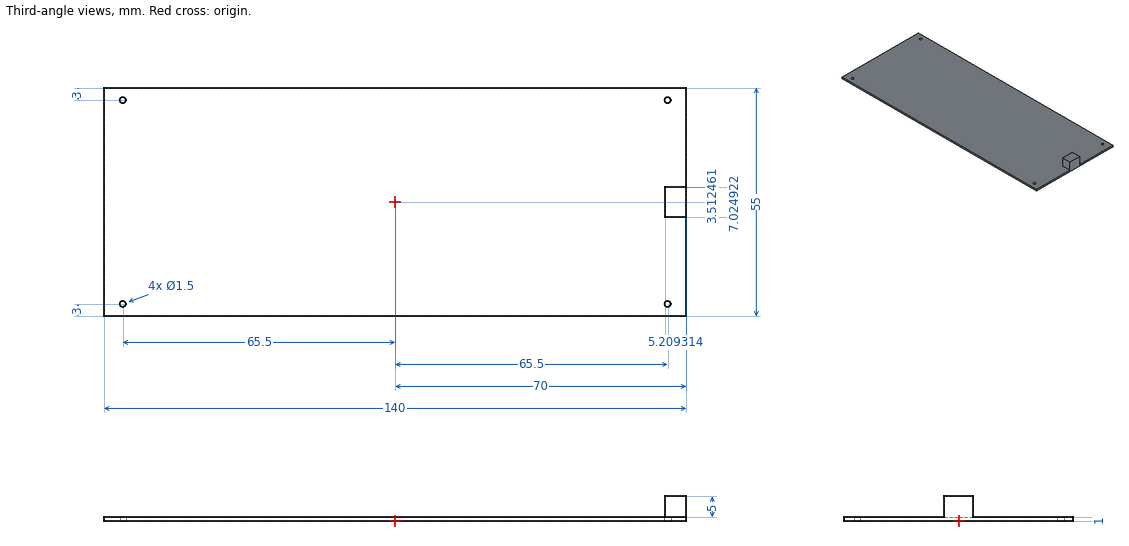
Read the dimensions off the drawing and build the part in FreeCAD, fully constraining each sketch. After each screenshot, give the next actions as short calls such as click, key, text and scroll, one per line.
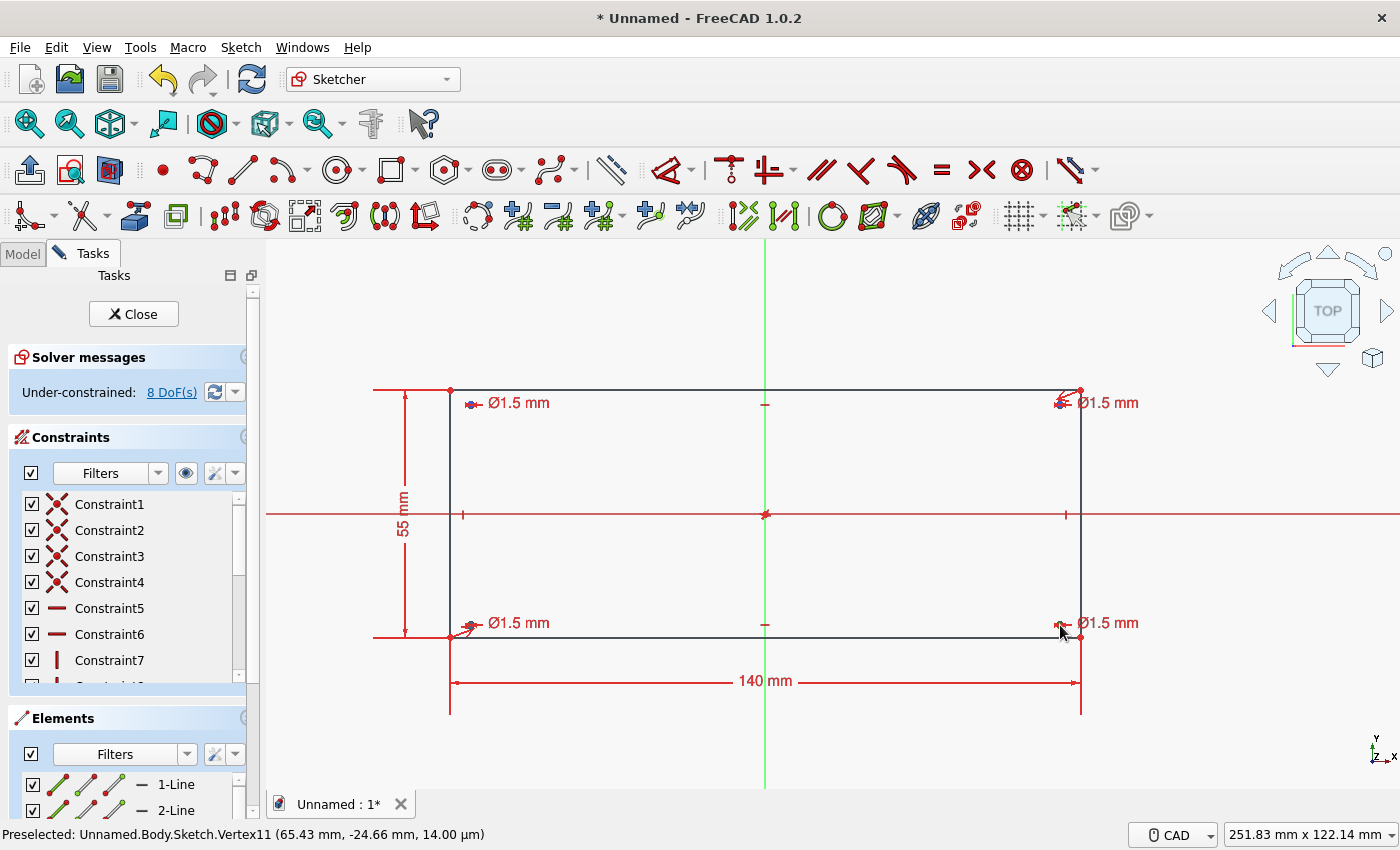
click(796, 170)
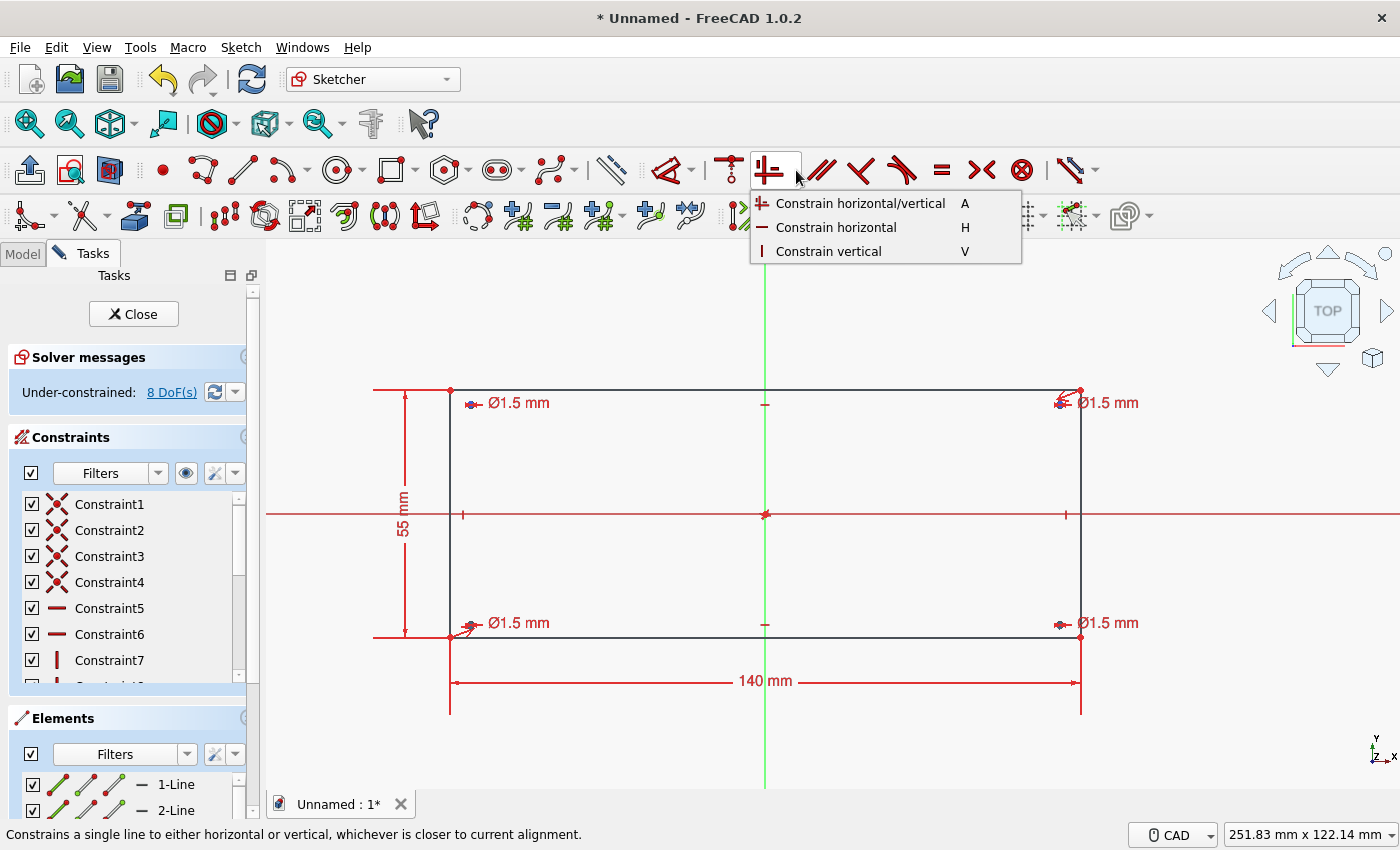
click(886, 227)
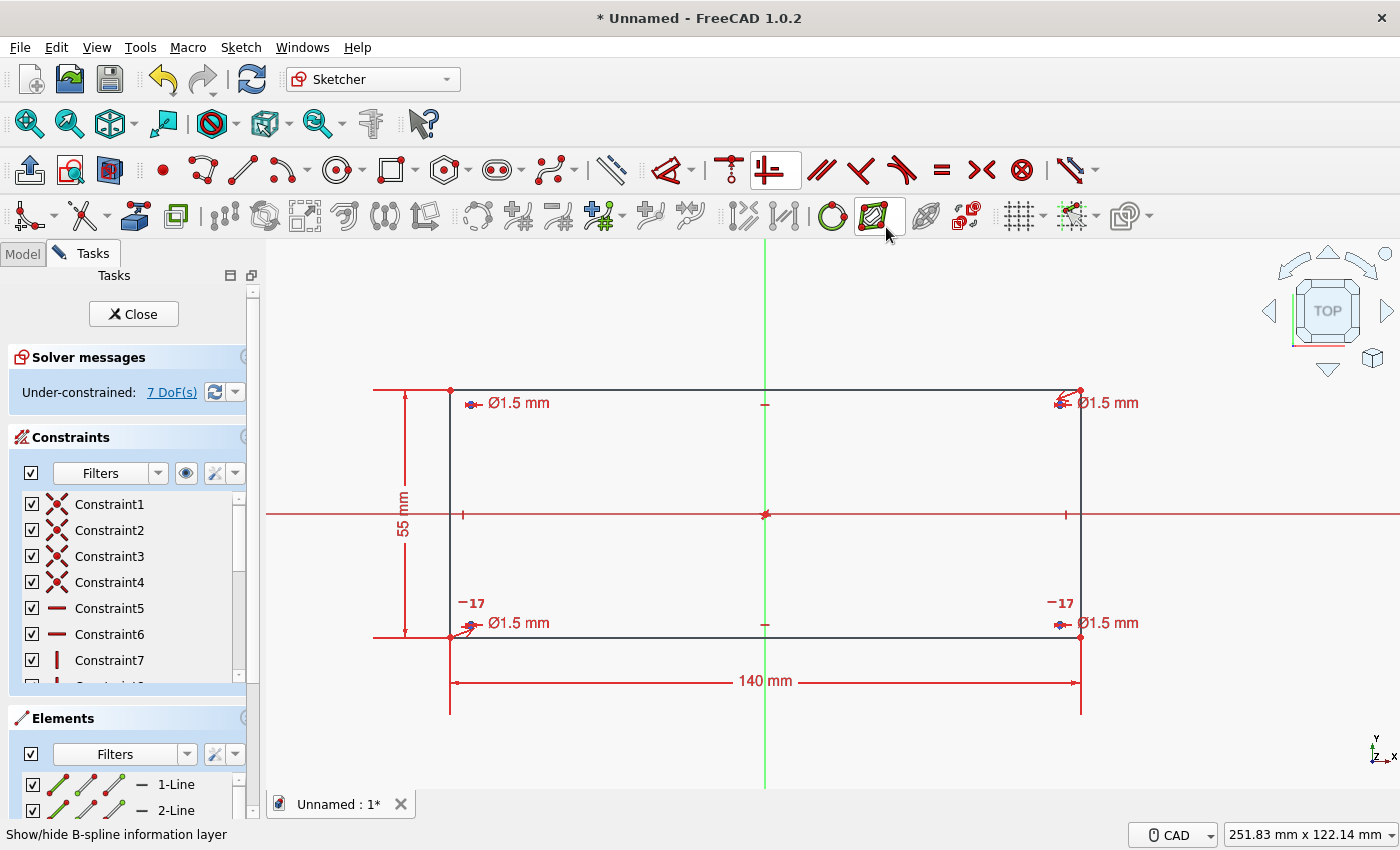
click(471, 625)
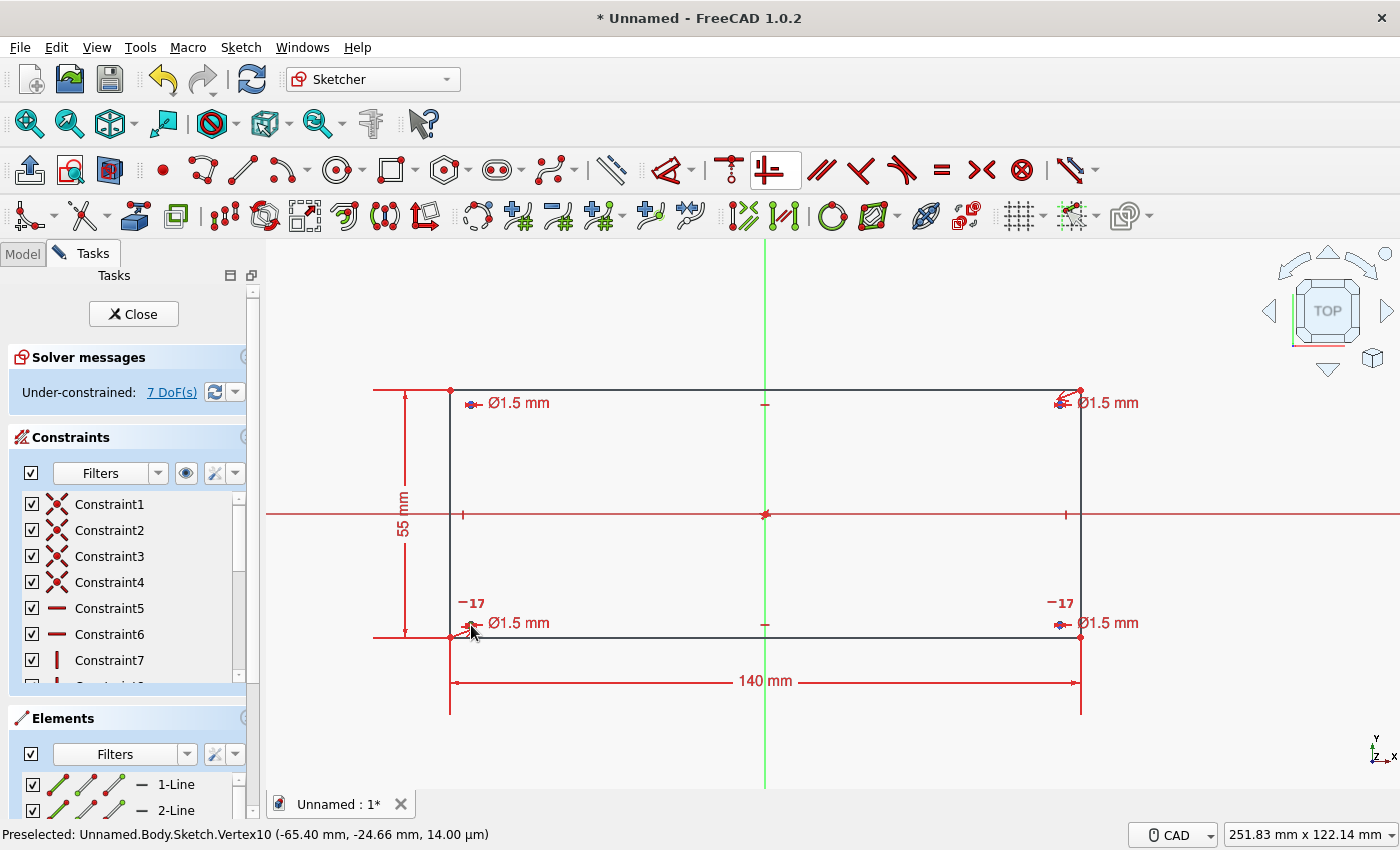
click(471, 405)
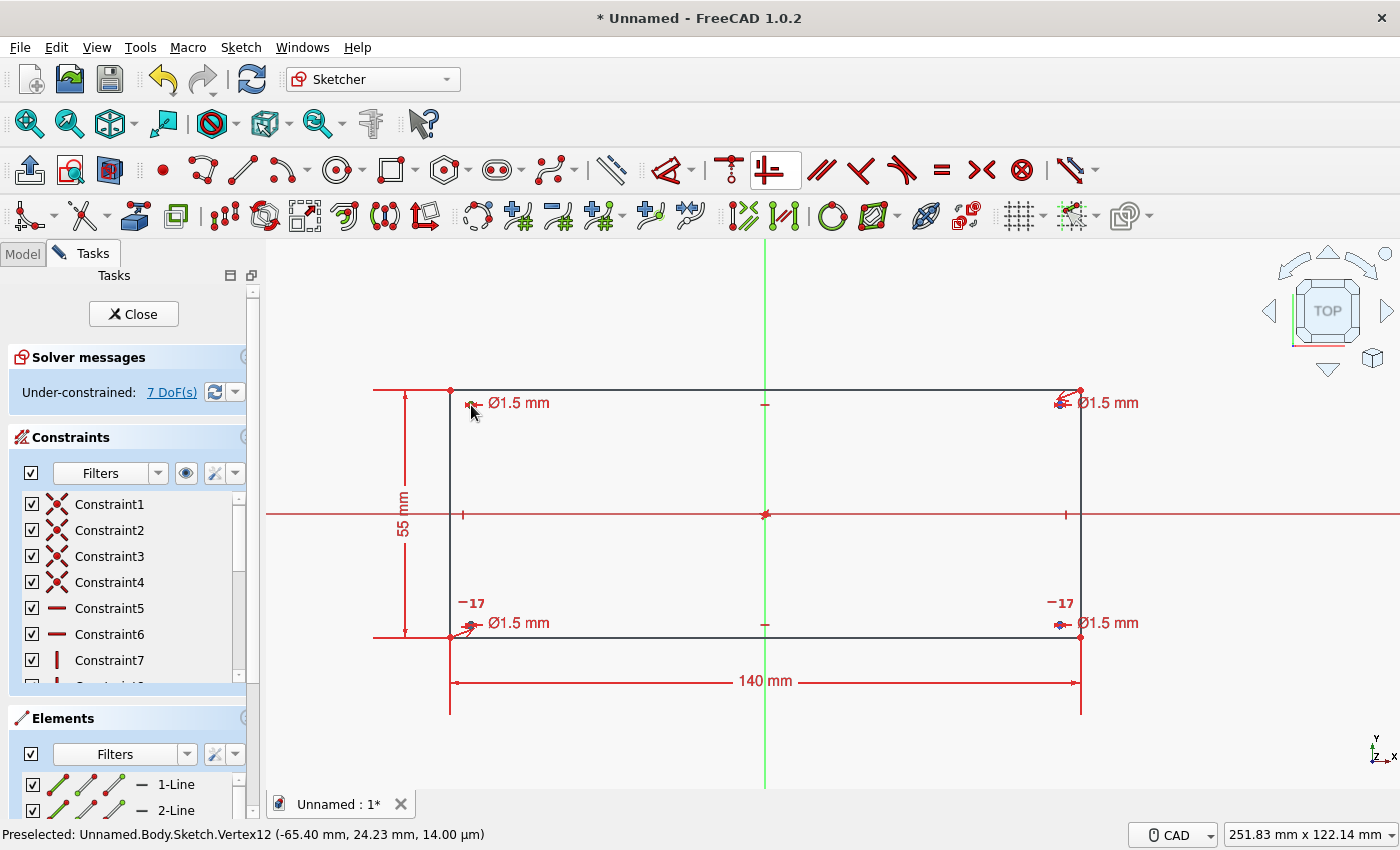
key(v)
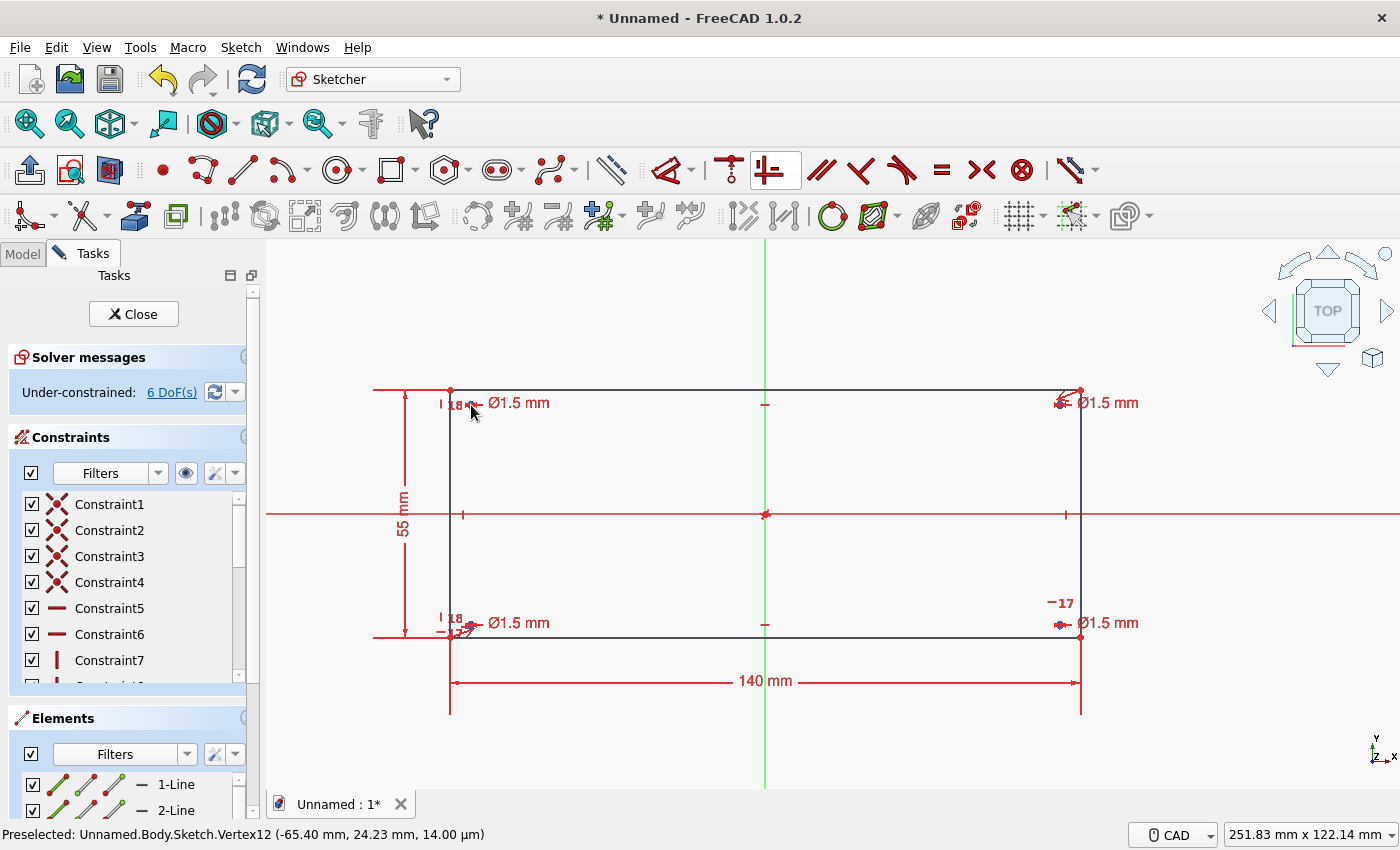
click(1060, 625)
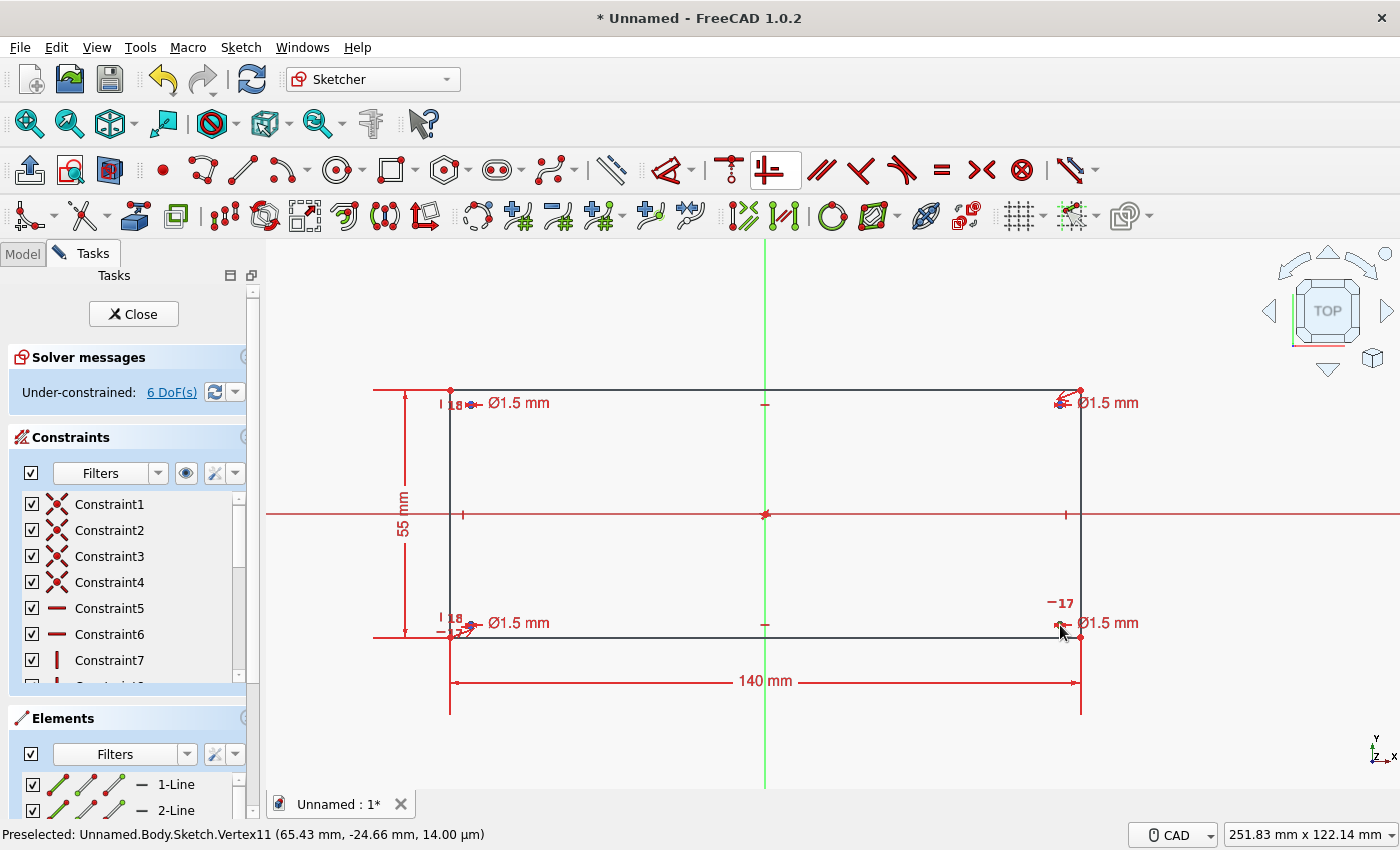
click(1060, 405)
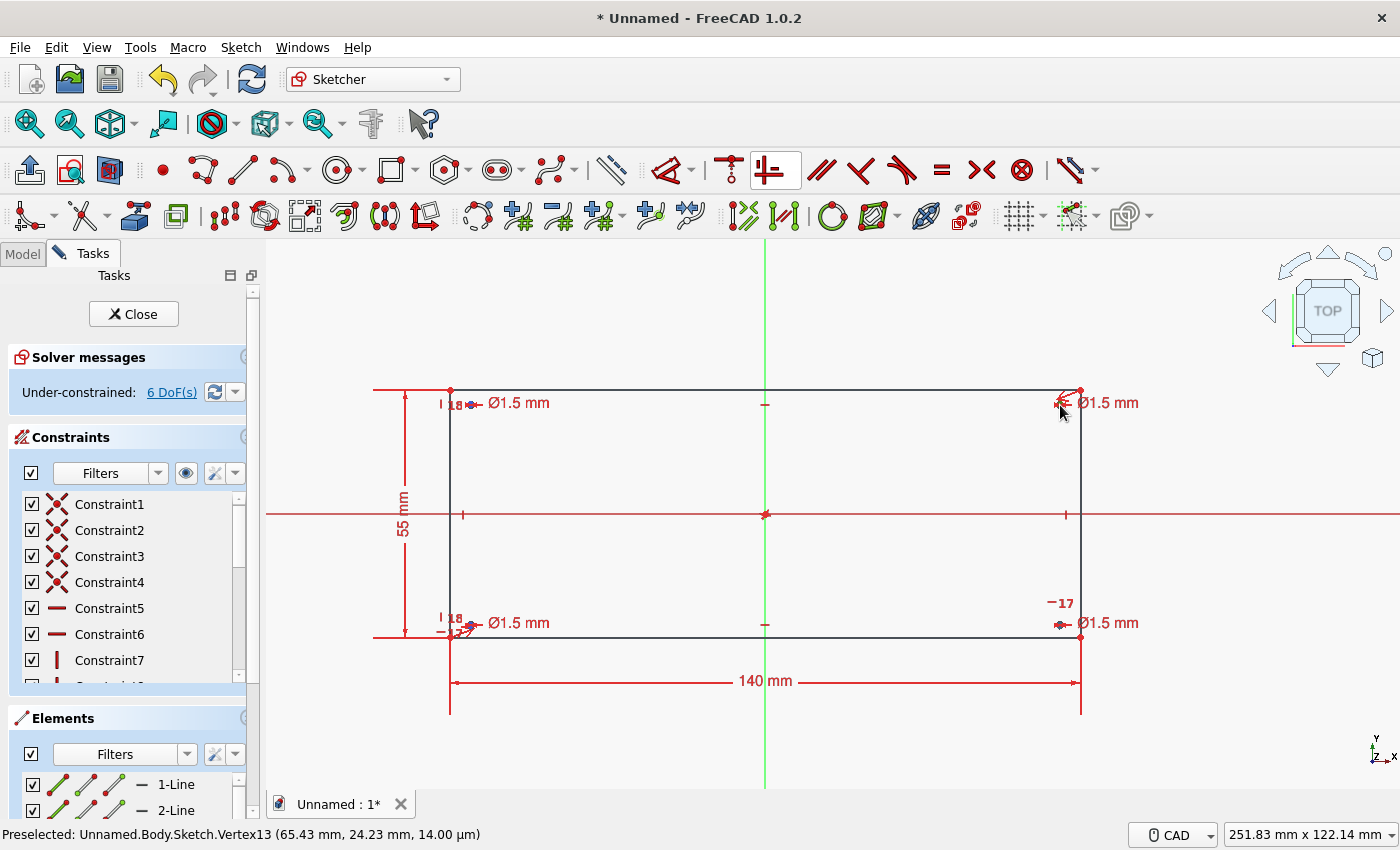
key(v)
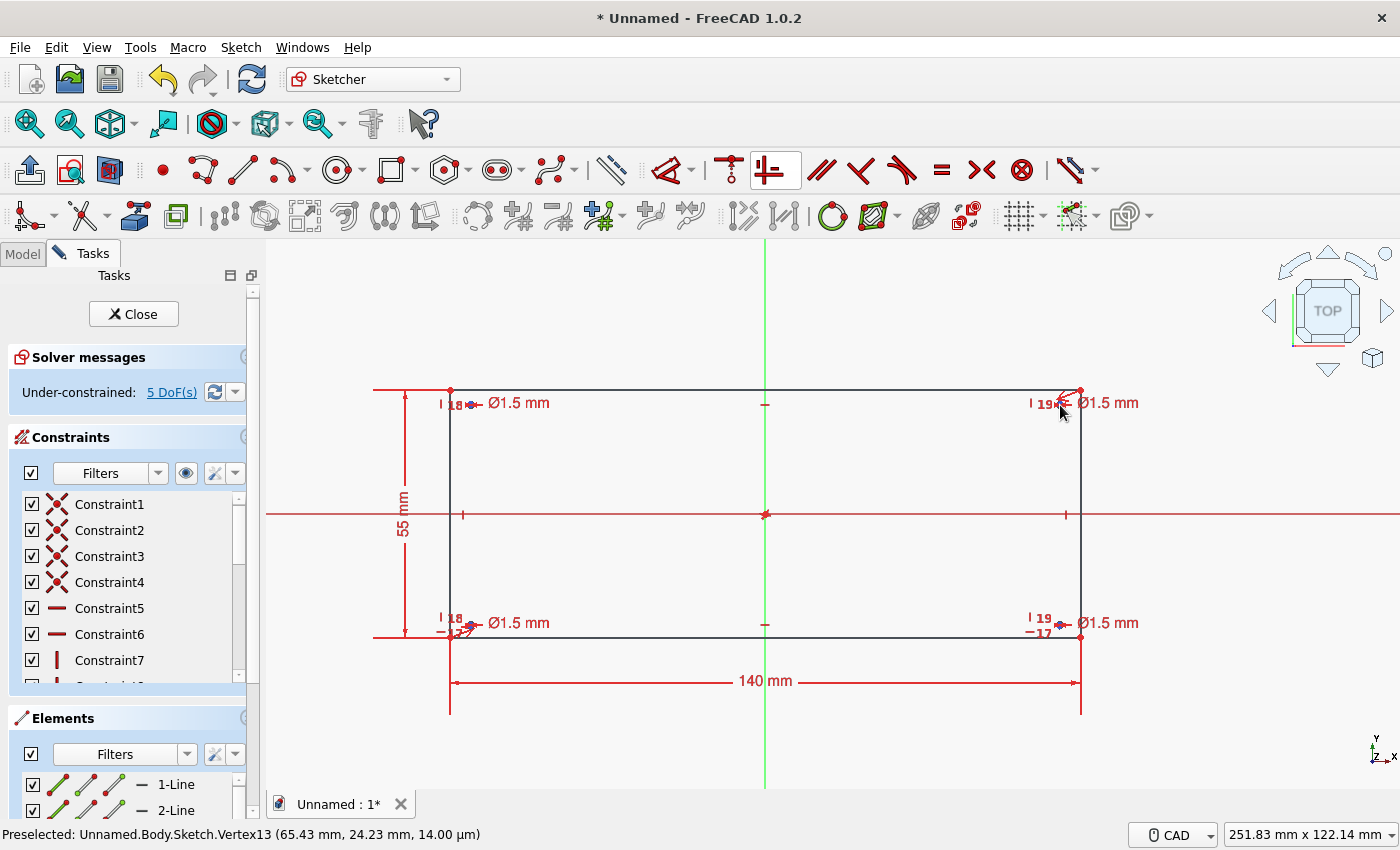
click(471, 405)